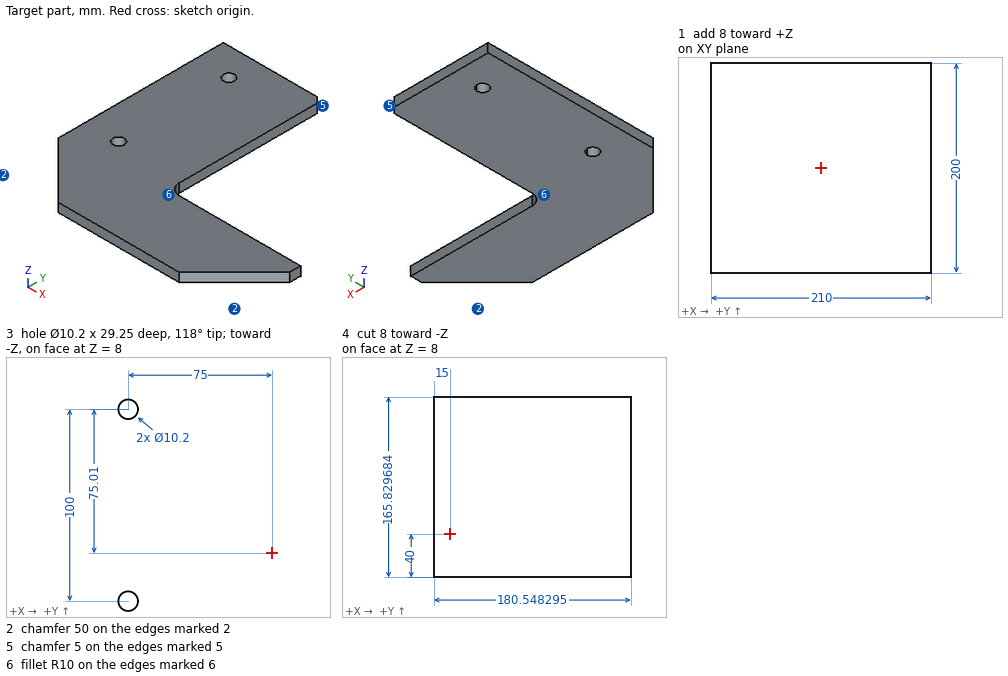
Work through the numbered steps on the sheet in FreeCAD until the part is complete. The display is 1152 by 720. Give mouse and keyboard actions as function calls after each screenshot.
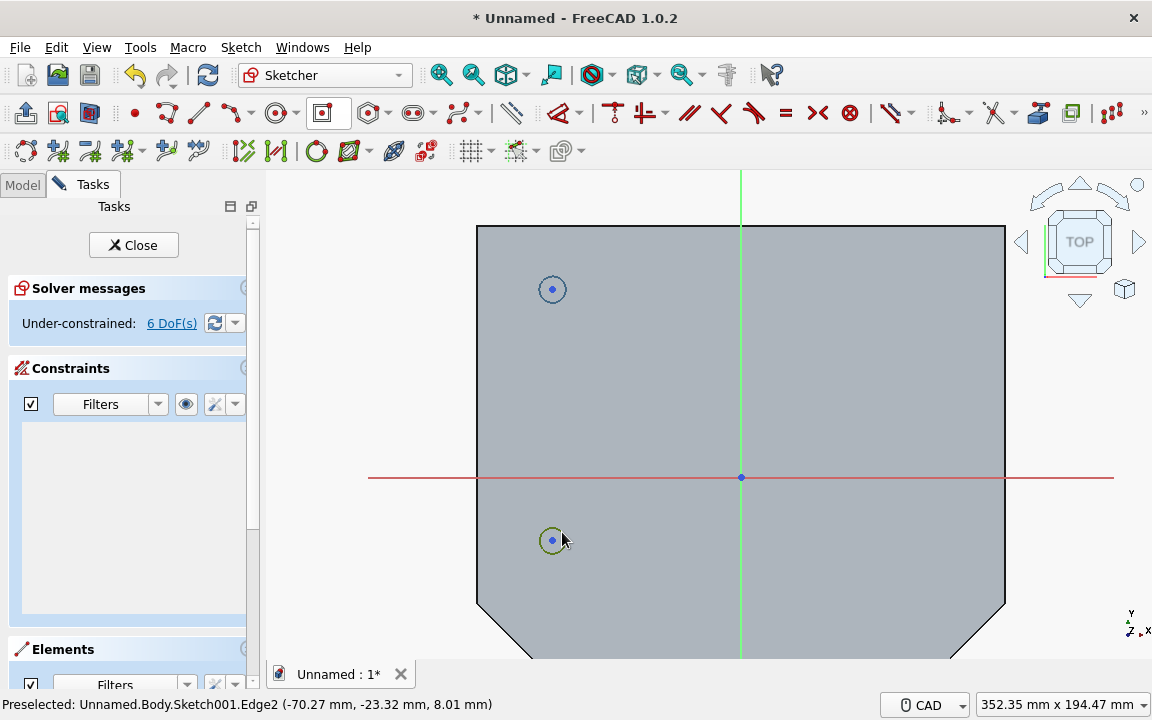
key(e)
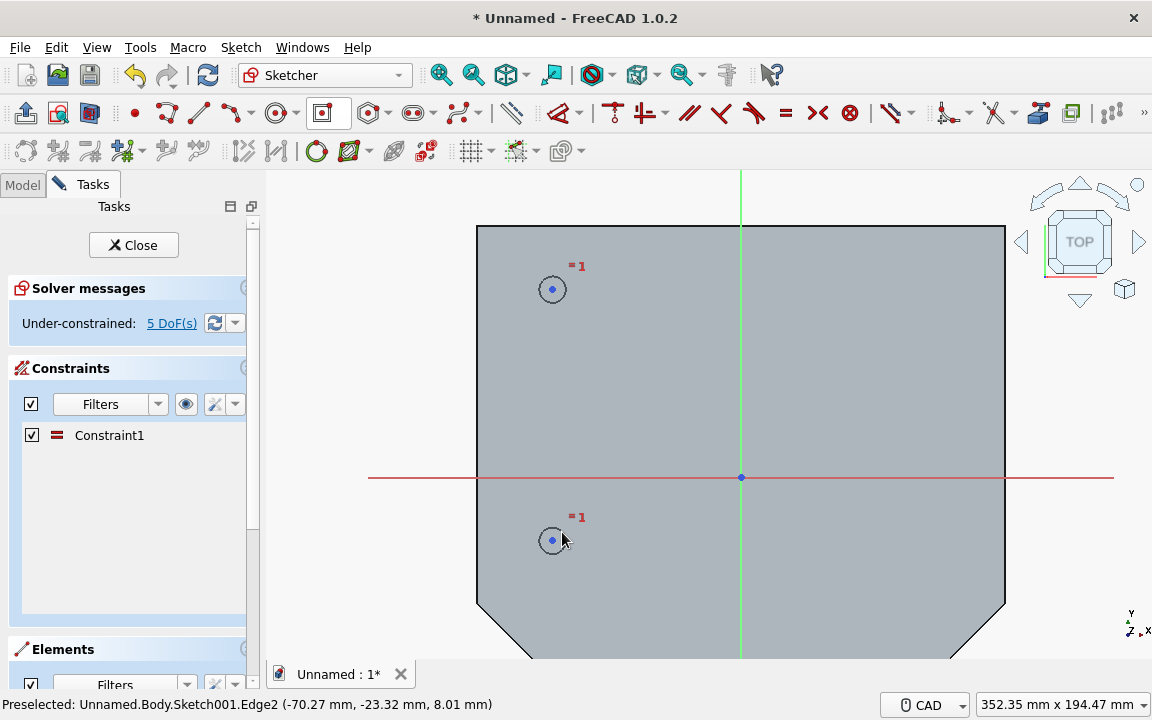
click(553, 290)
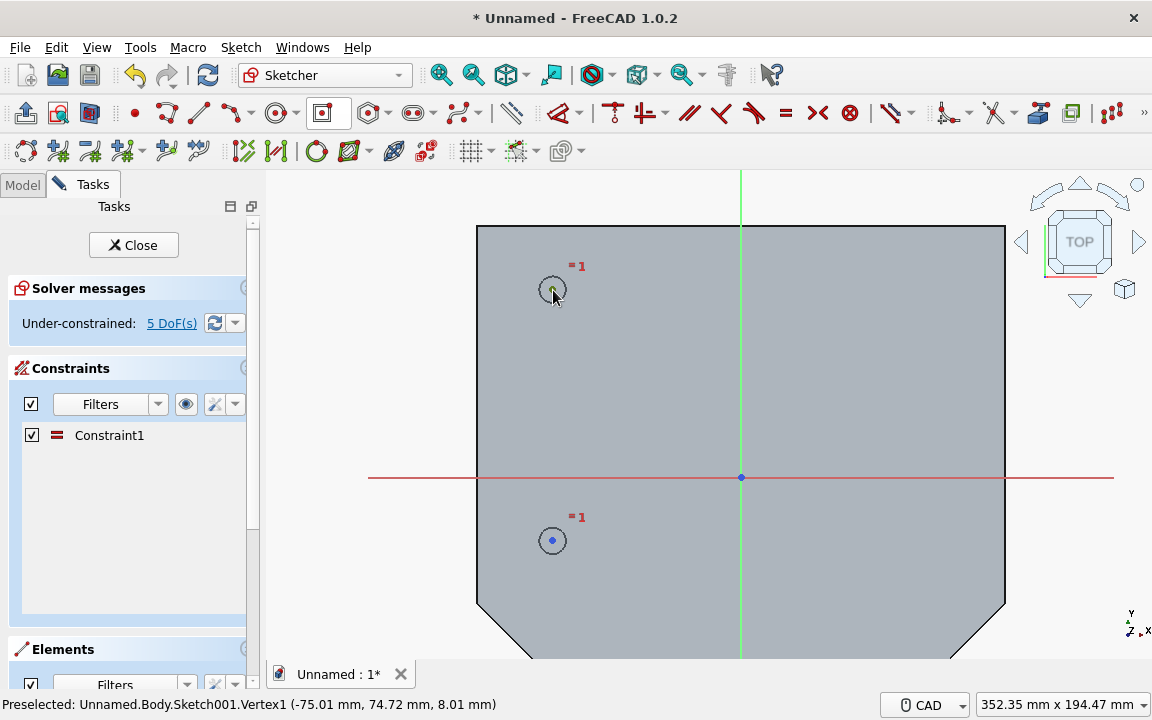
click(553, 541)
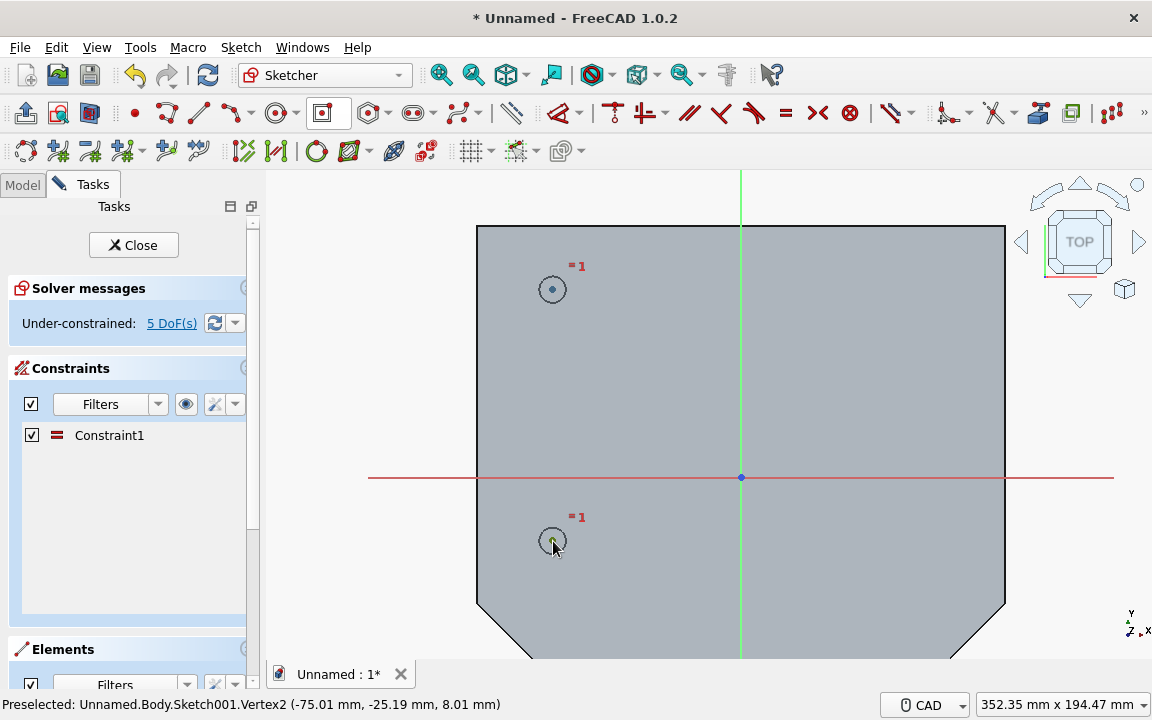
click(668, 114)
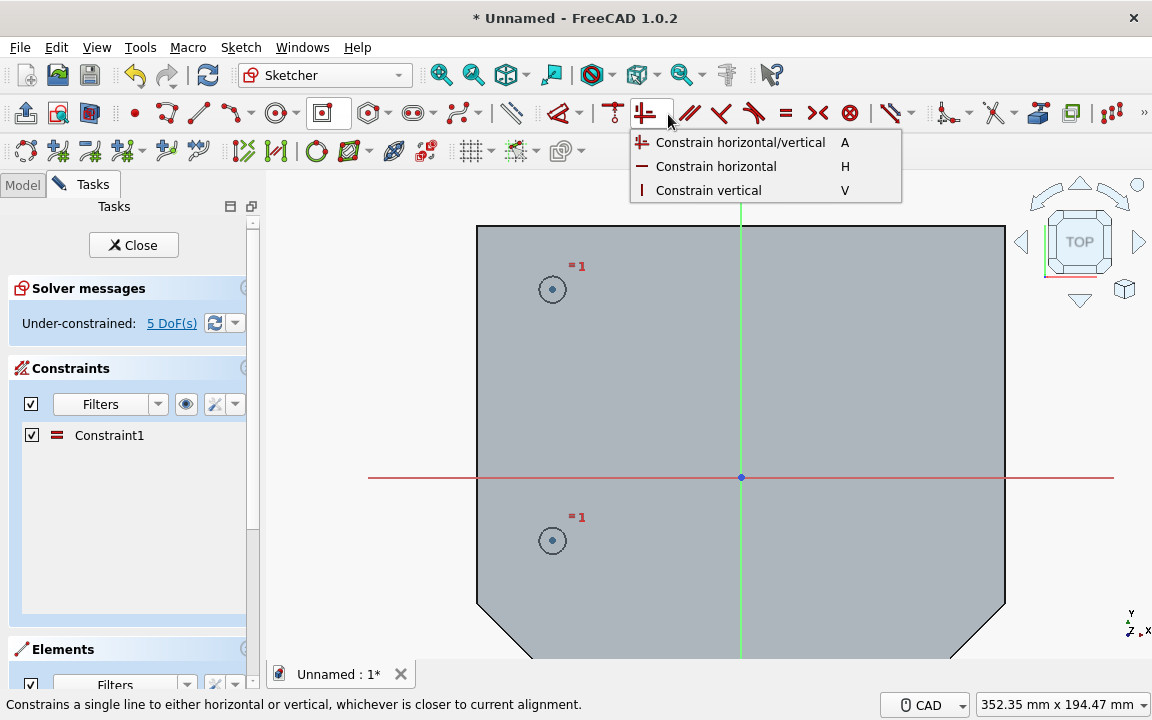
click(766, 190)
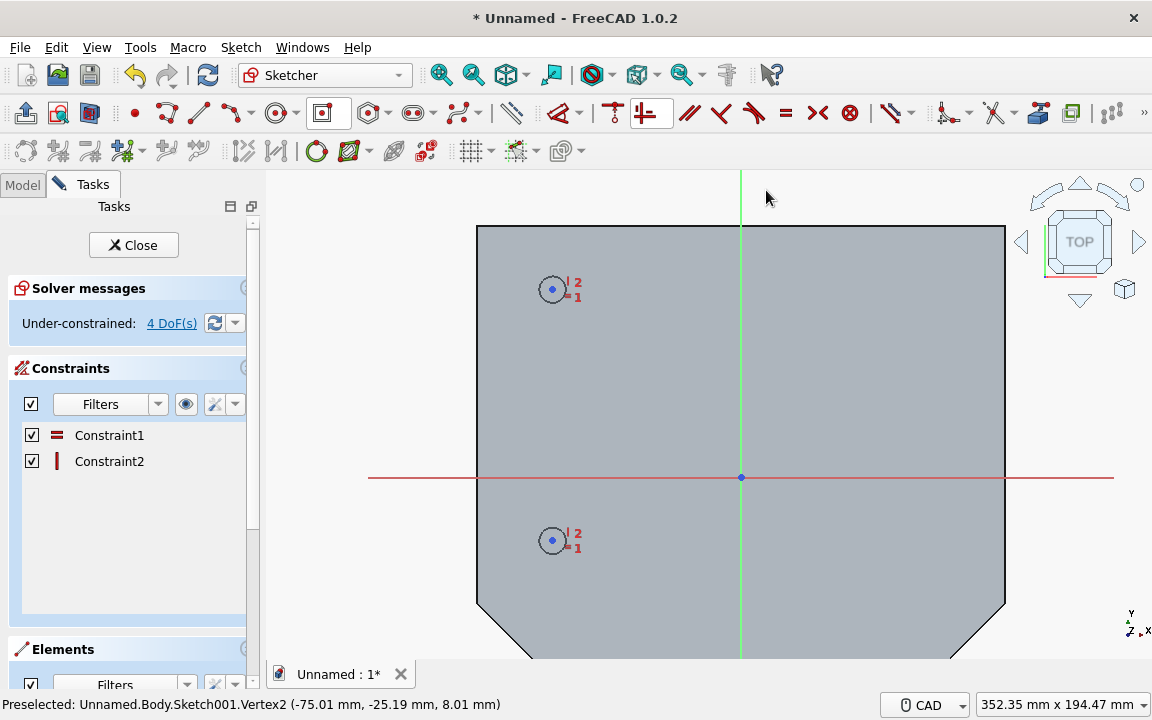
scroll(562, 280, up, 3)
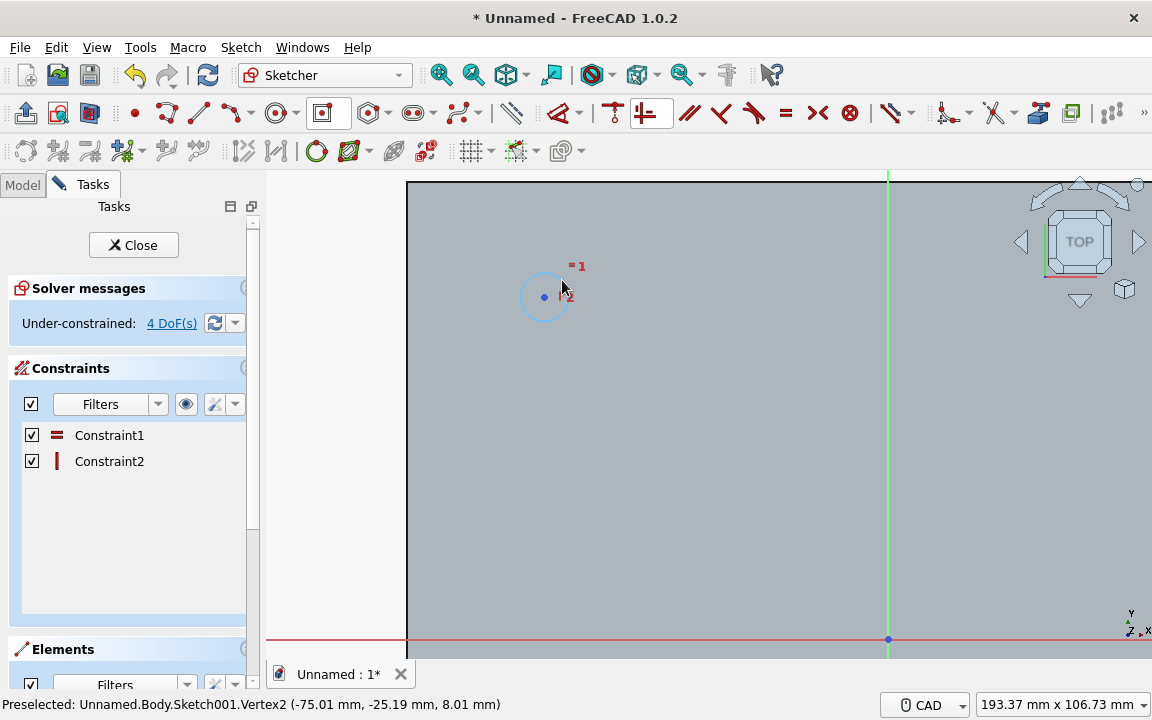
click(562, 280)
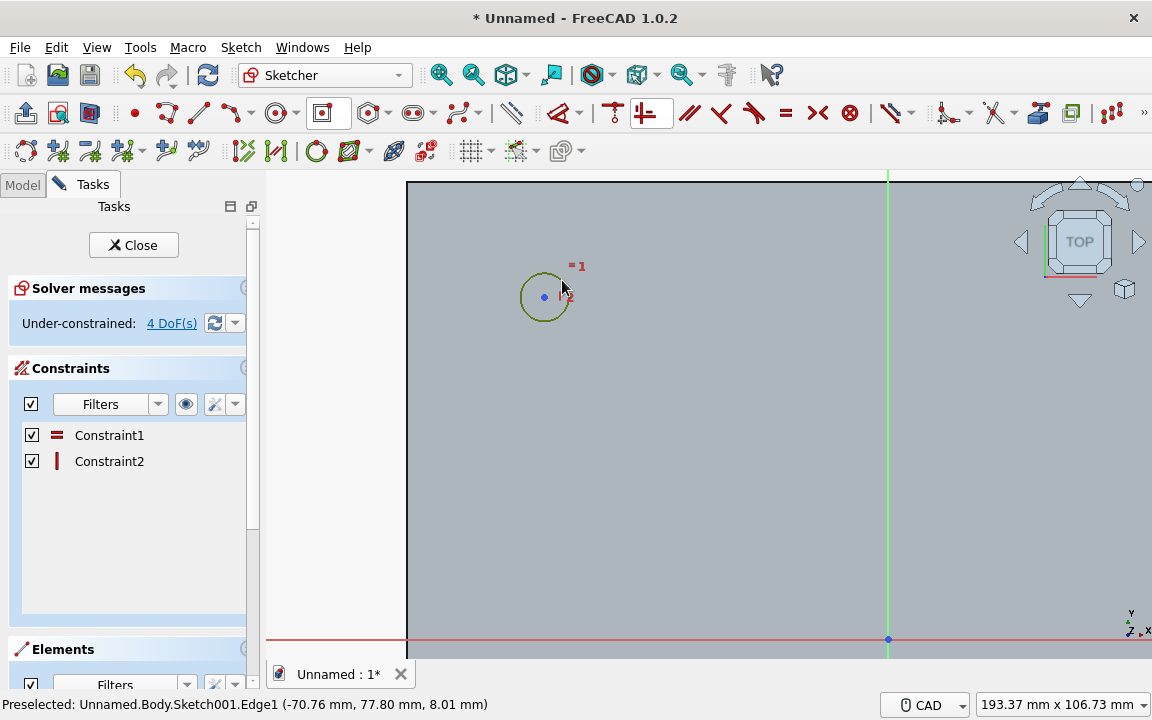
key(k)
key(o)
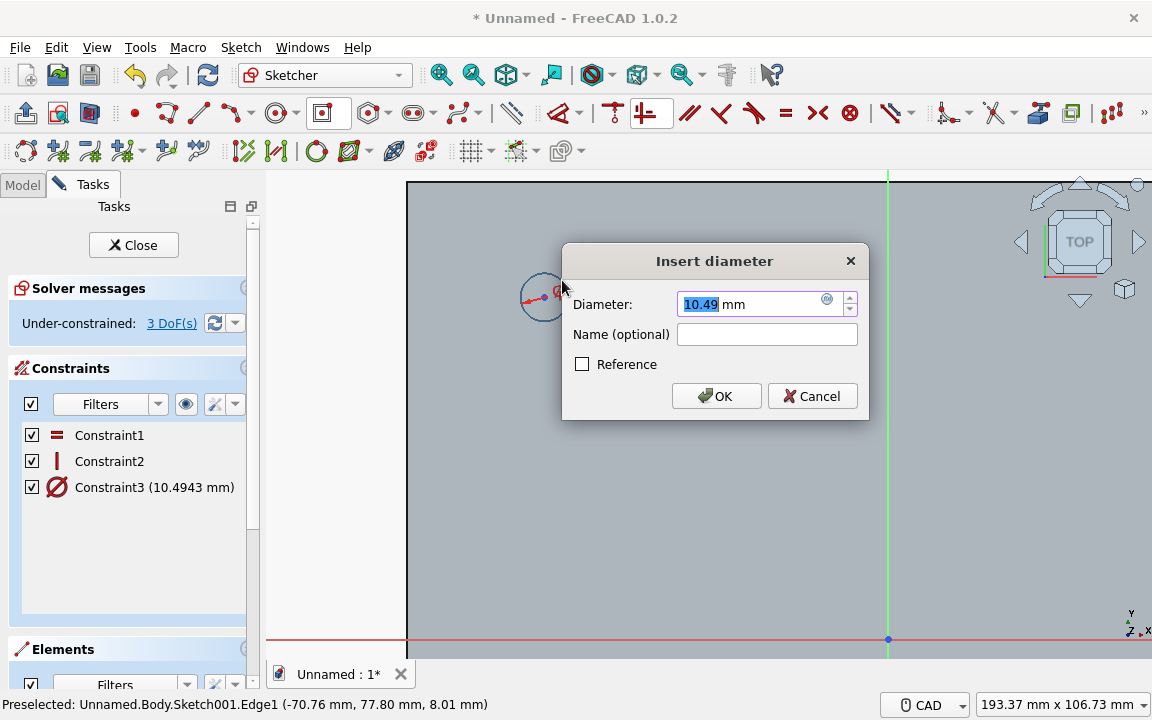
text(10.2)
key(Return)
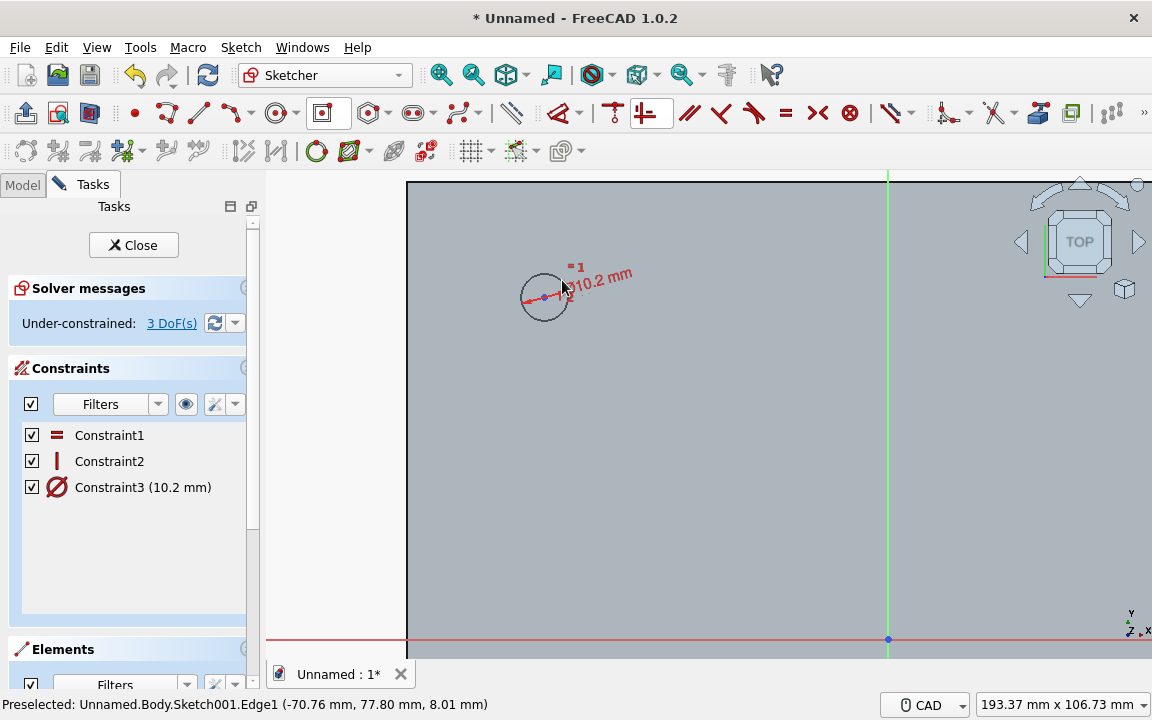
click(545, 297)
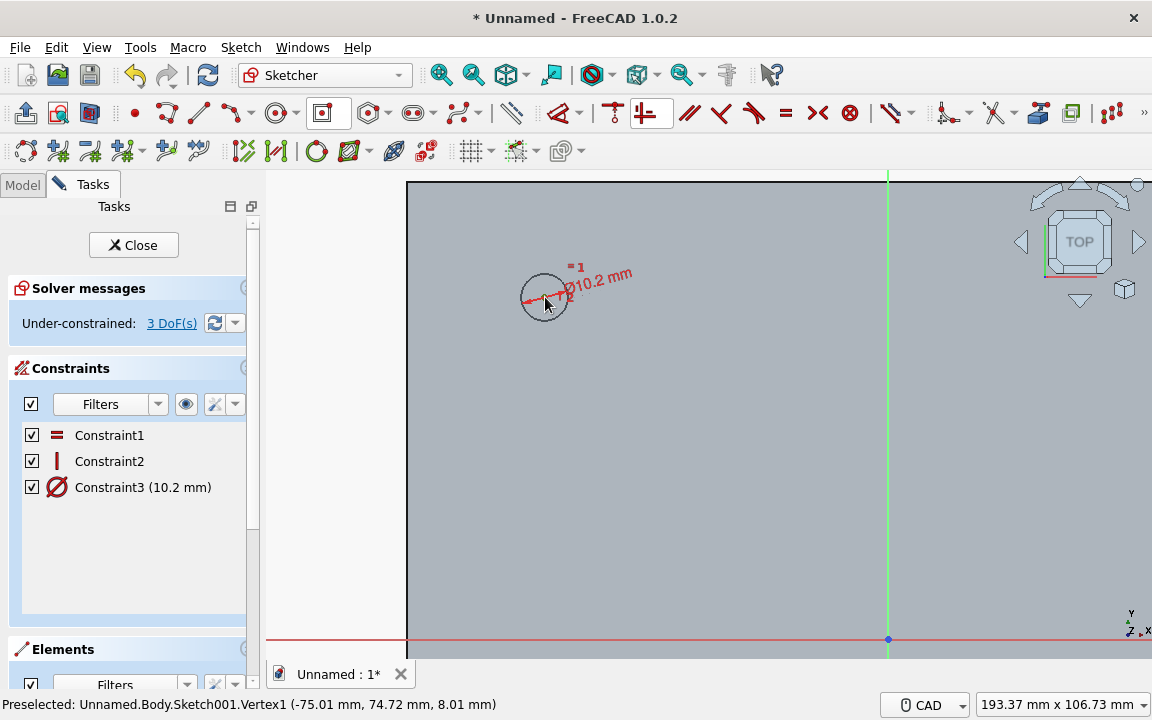
key(l)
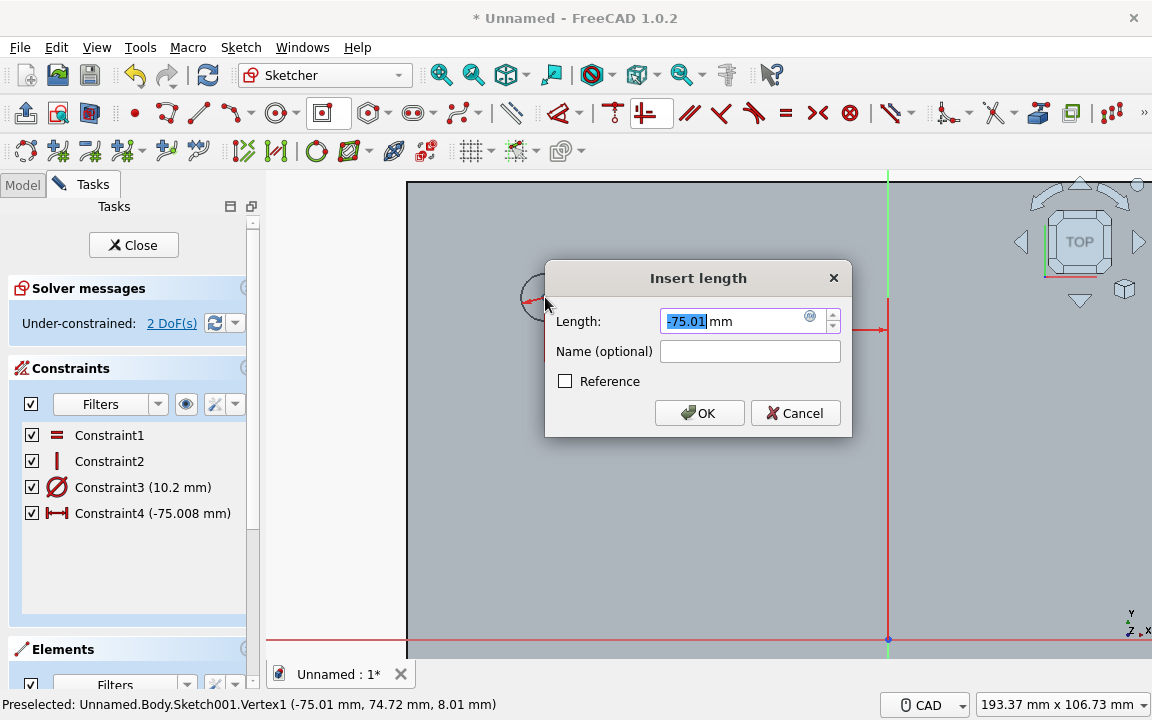
text(-75)
key(Return)